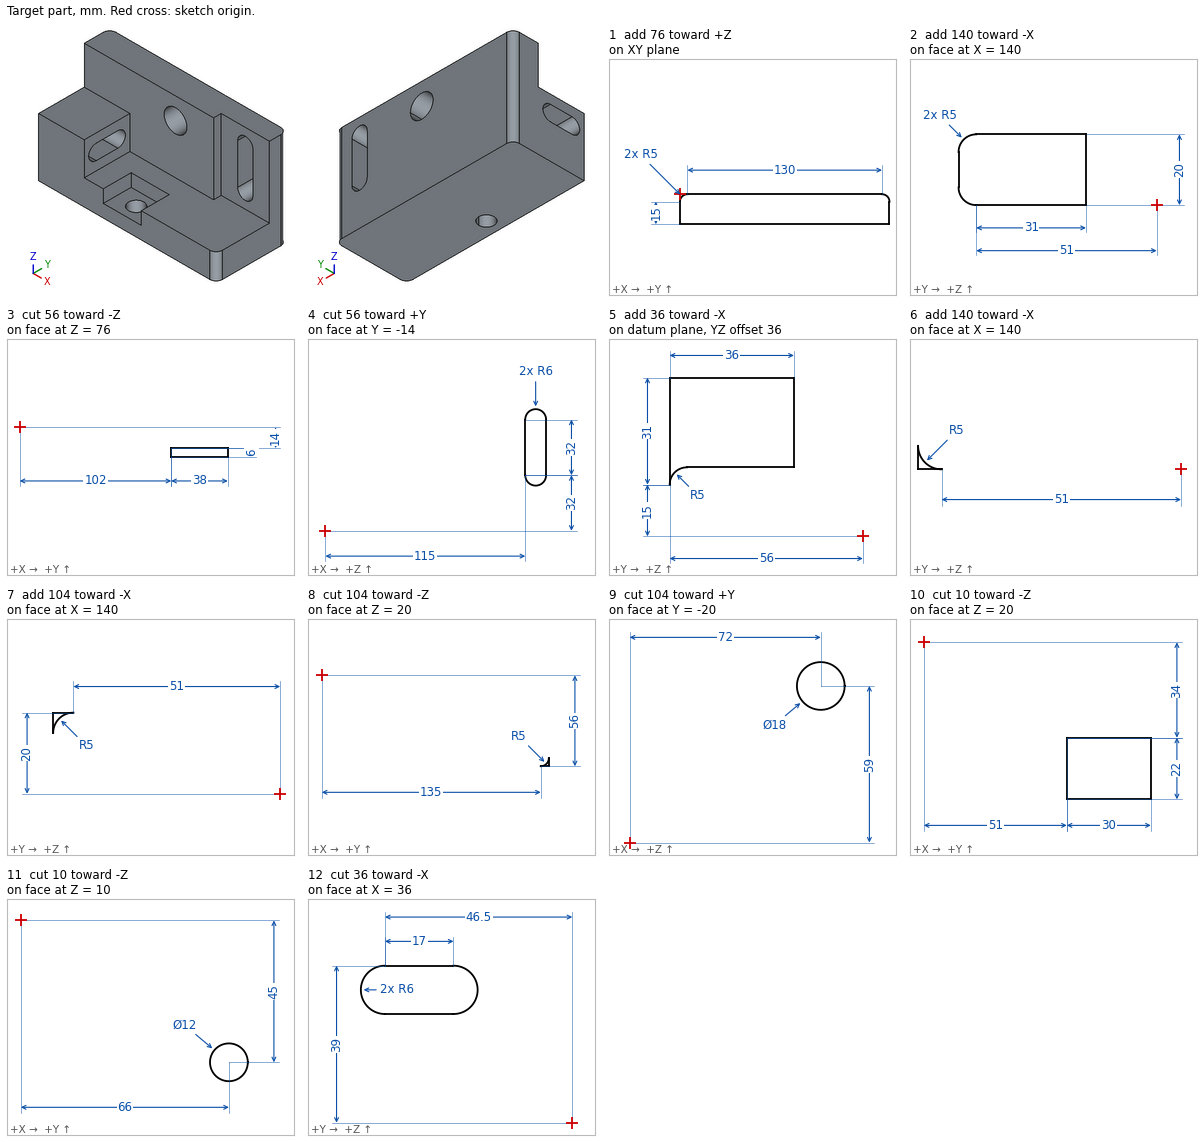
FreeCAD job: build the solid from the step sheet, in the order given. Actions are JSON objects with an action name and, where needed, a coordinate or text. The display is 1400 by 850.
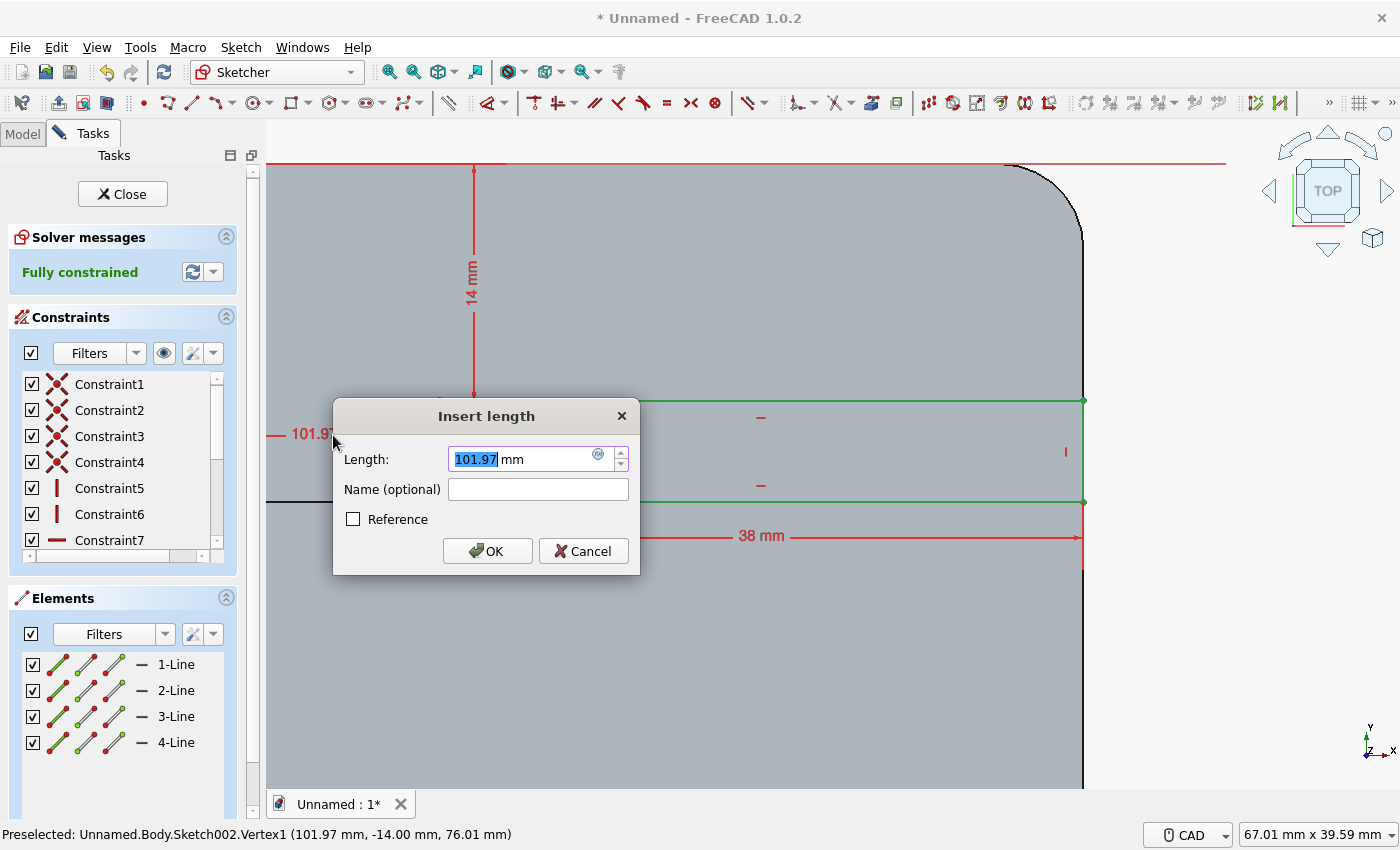
{"action": "type", "text": "102"}
{"action": "key", "text": "Return"}
{"action": "key", "text": "Escape"}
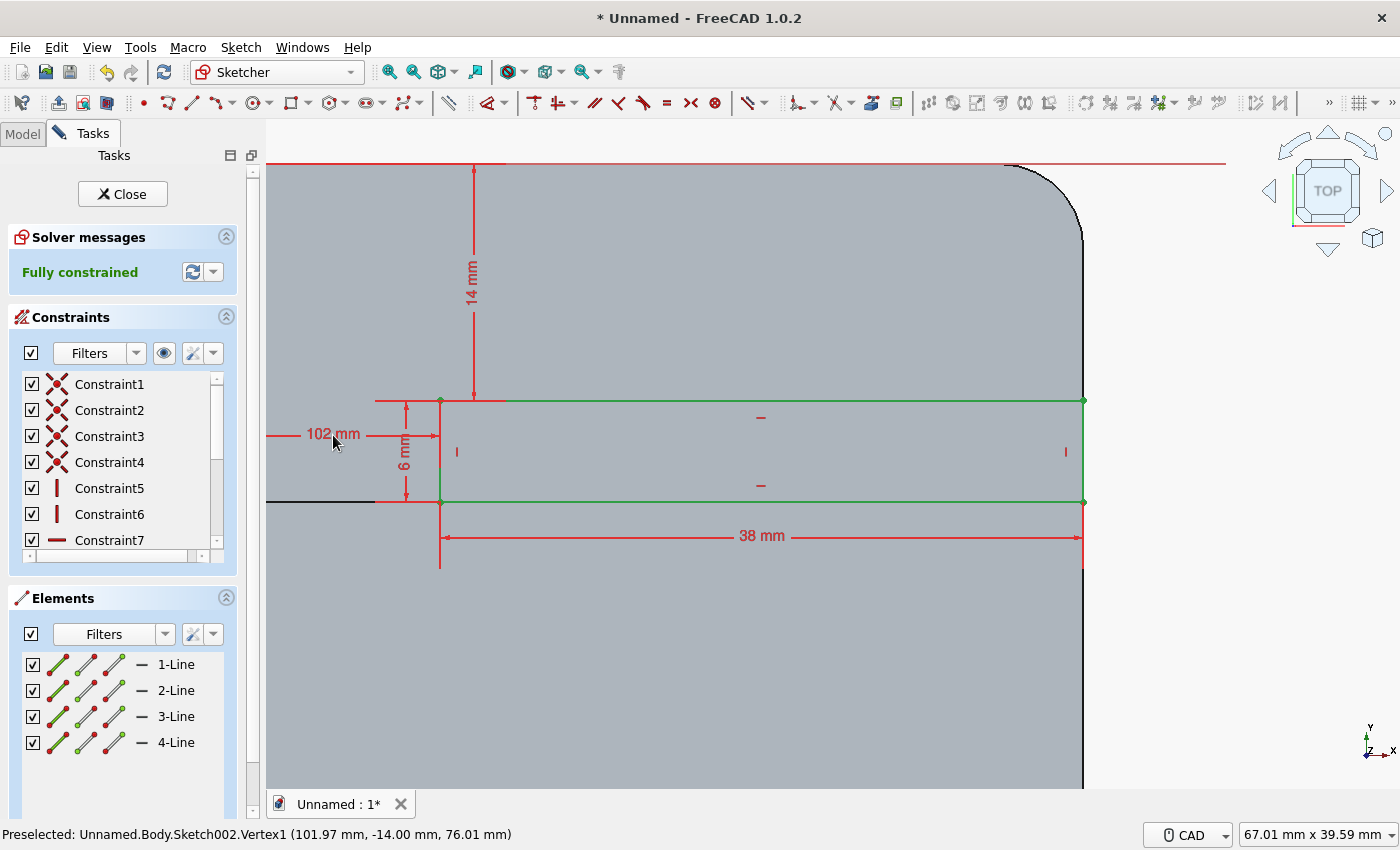
{"action": "left_click", "coordinate": [123, 194]}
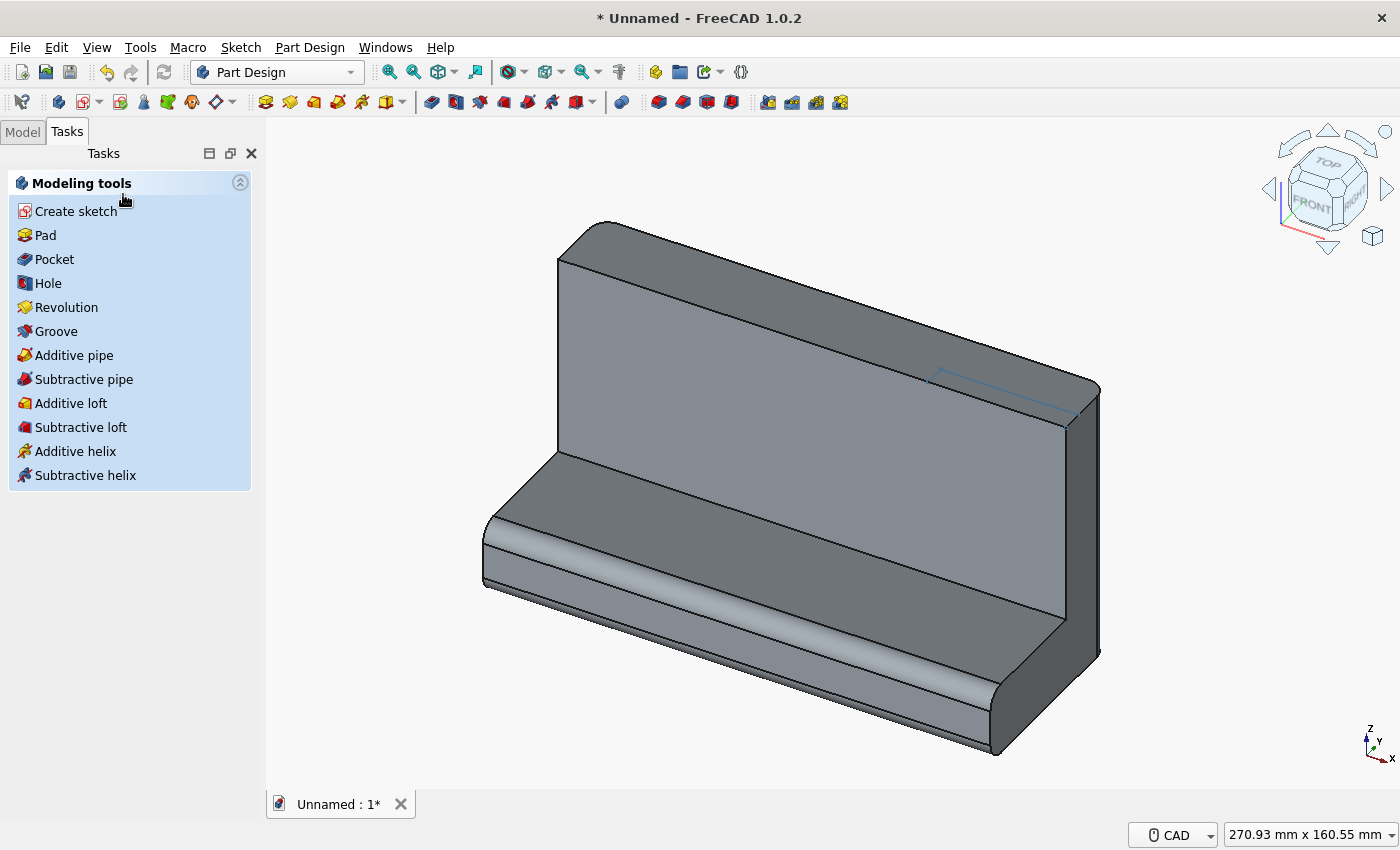
{"action": "left_click", "coordinate": [432, 102]}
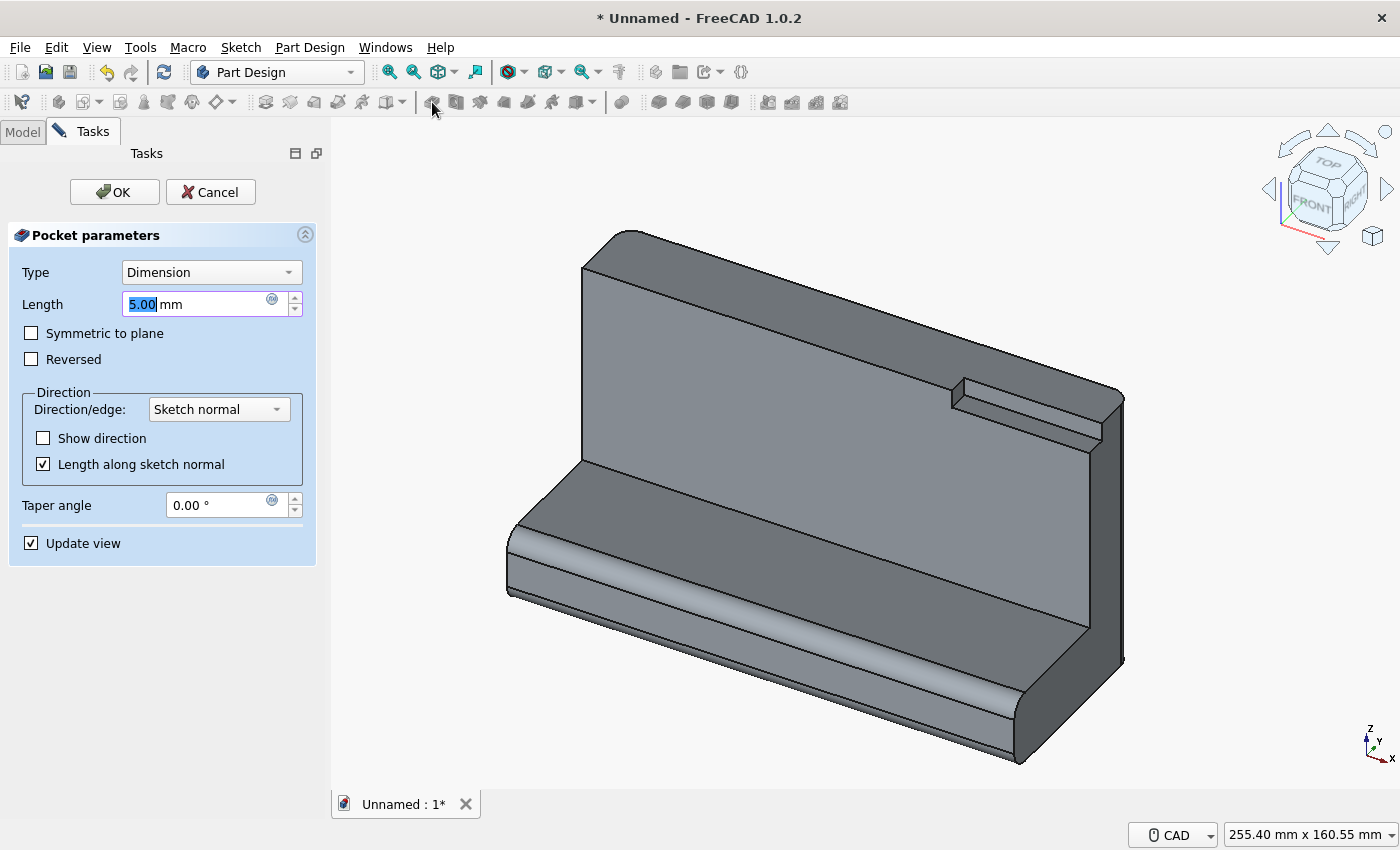
{"action": "type", "text": "56"}
{"action": "key", "text": "Tab"}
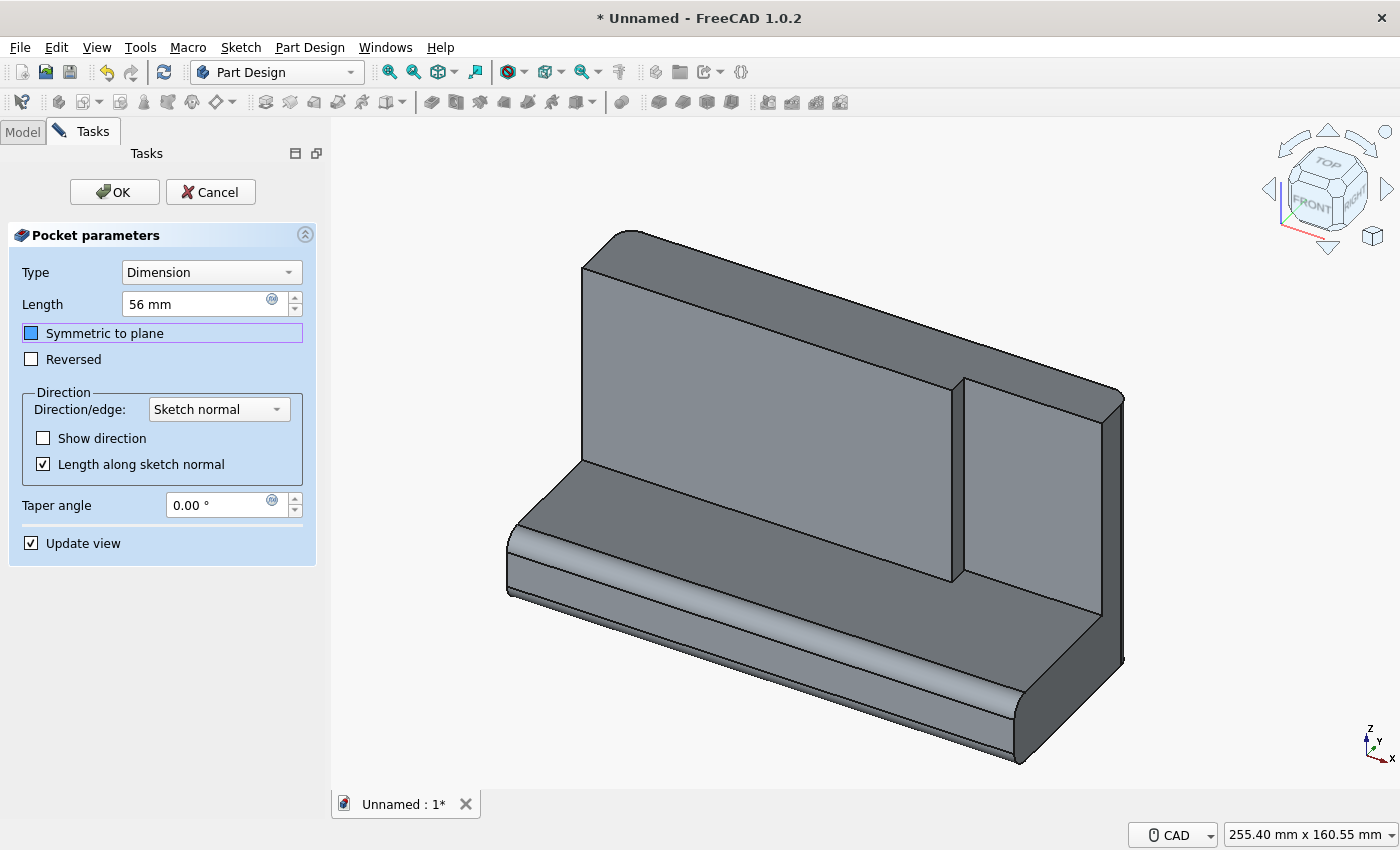
{"action": "left_click", "coordinate": [115, 192]}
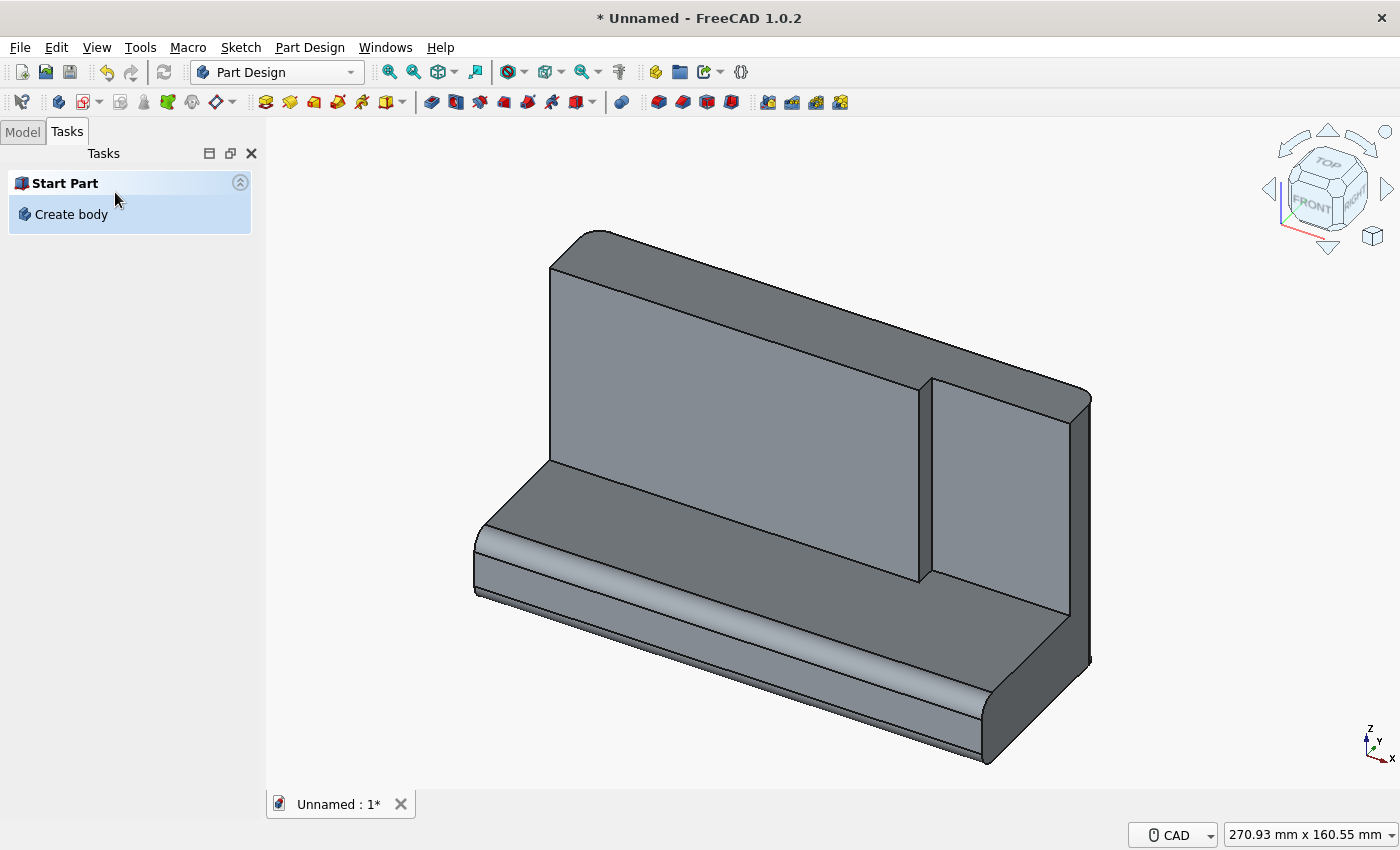
{"action": "left_click", "coordinate": [1001, 468]}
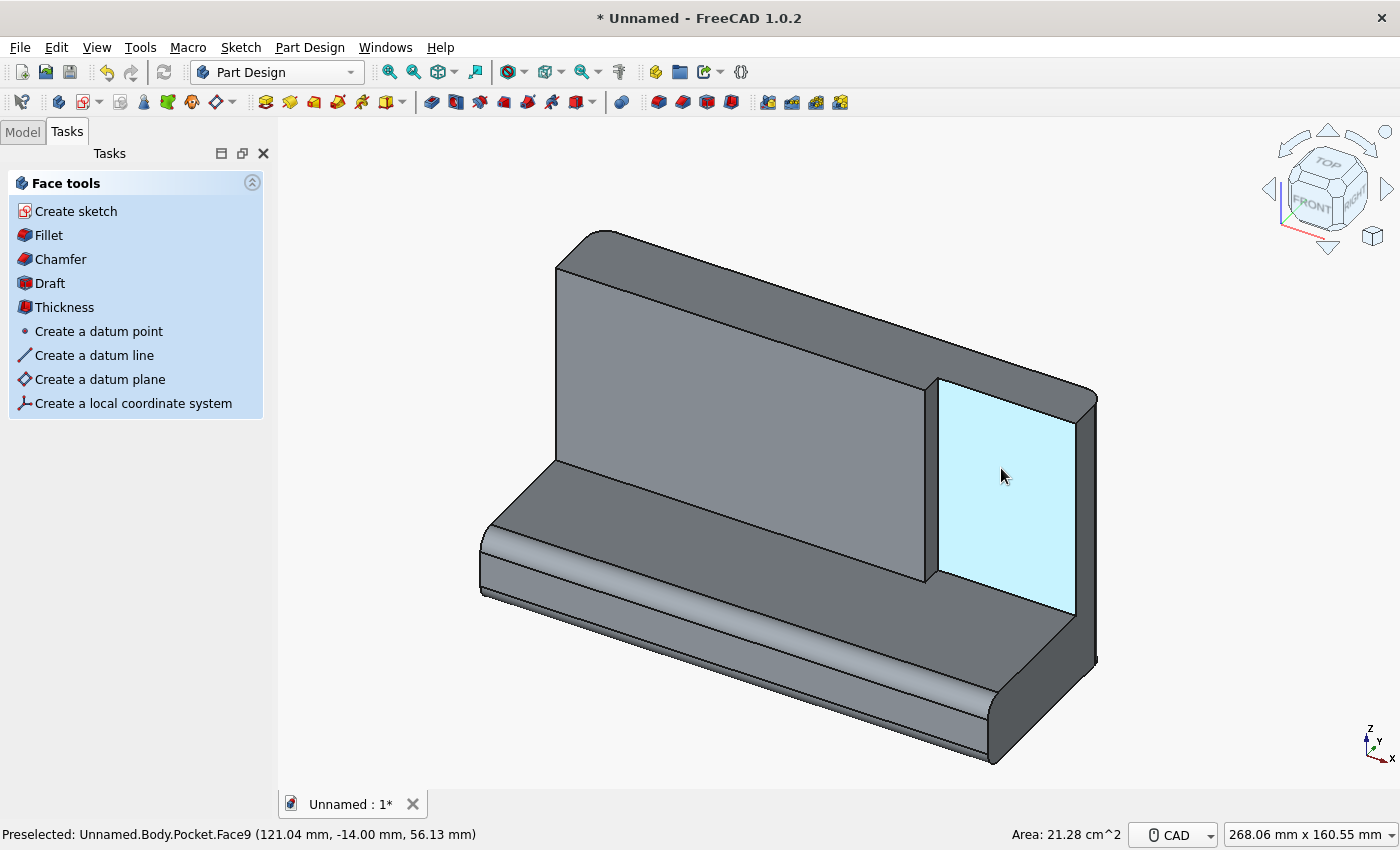
{"action": "left_click", "coordinate": [84, 102]}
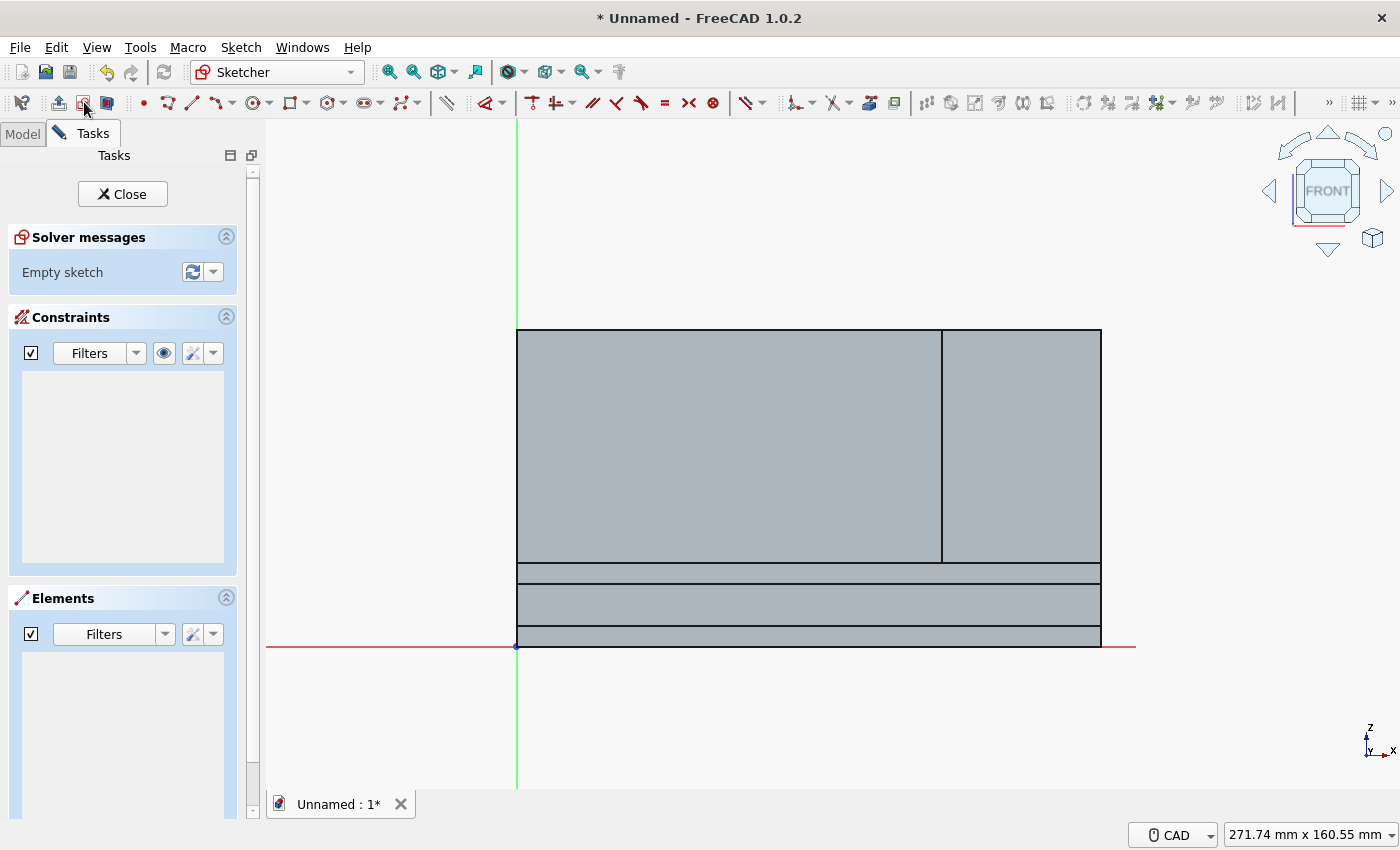
{"action": "left_click", "coordinate": [108, 104]}